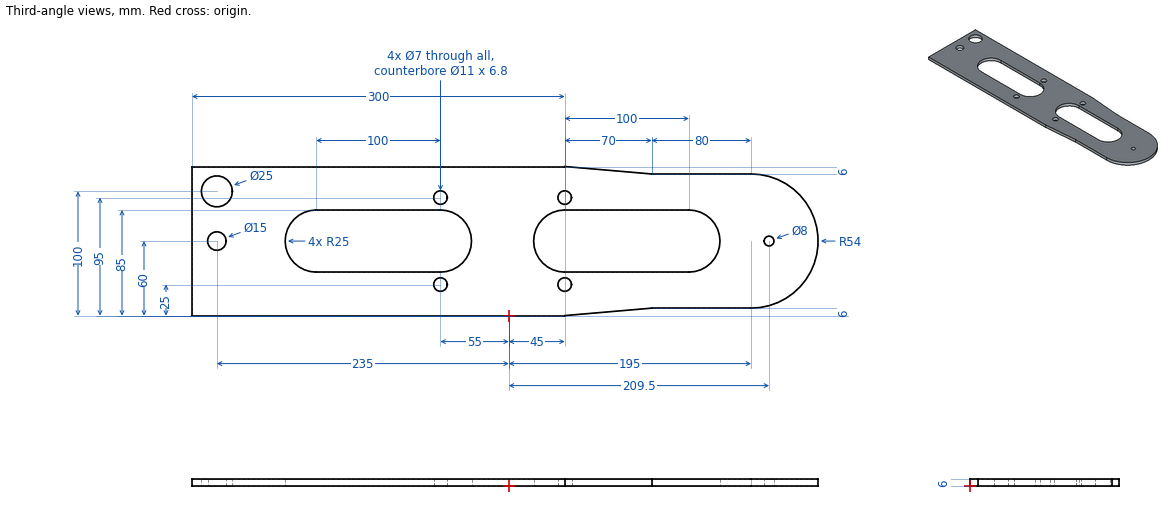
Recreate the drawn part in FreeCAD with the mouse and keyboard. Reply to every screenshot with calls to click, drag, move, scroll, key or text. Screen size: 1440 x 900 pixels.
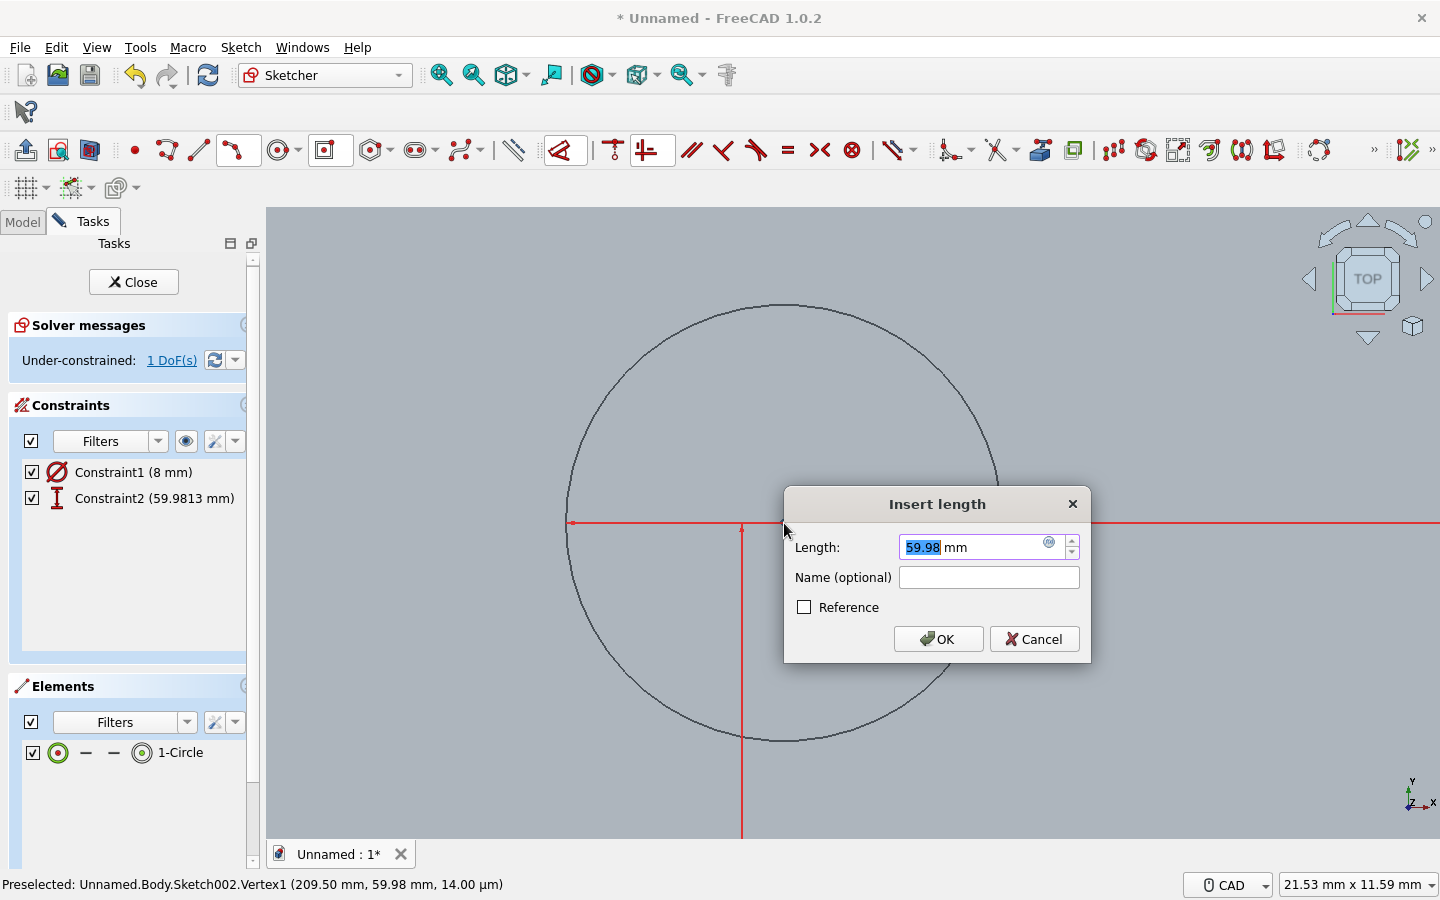
text(60)
key(Return)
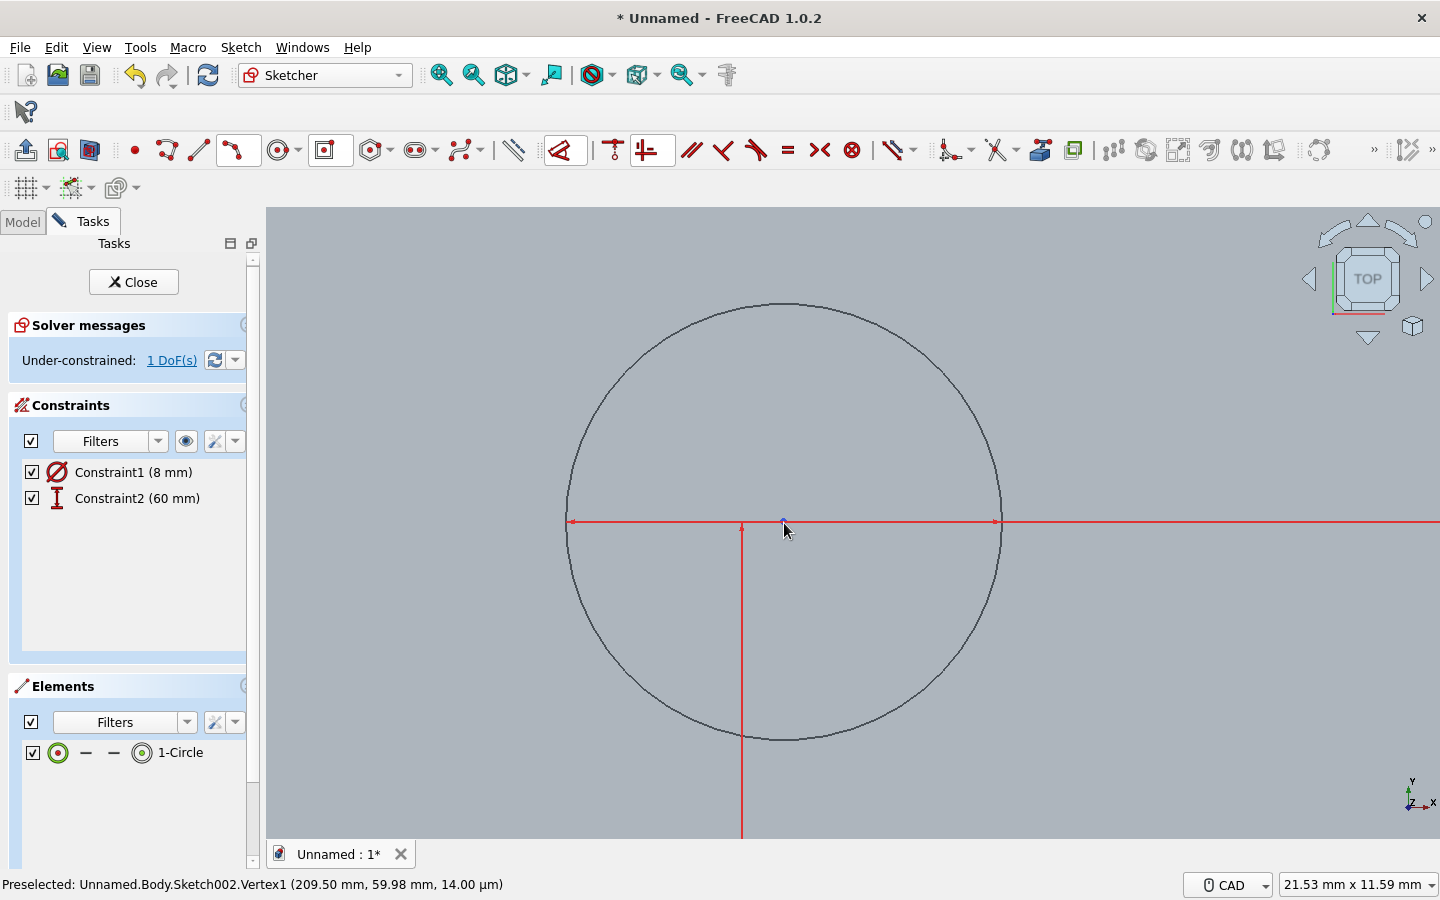
click(784, 522)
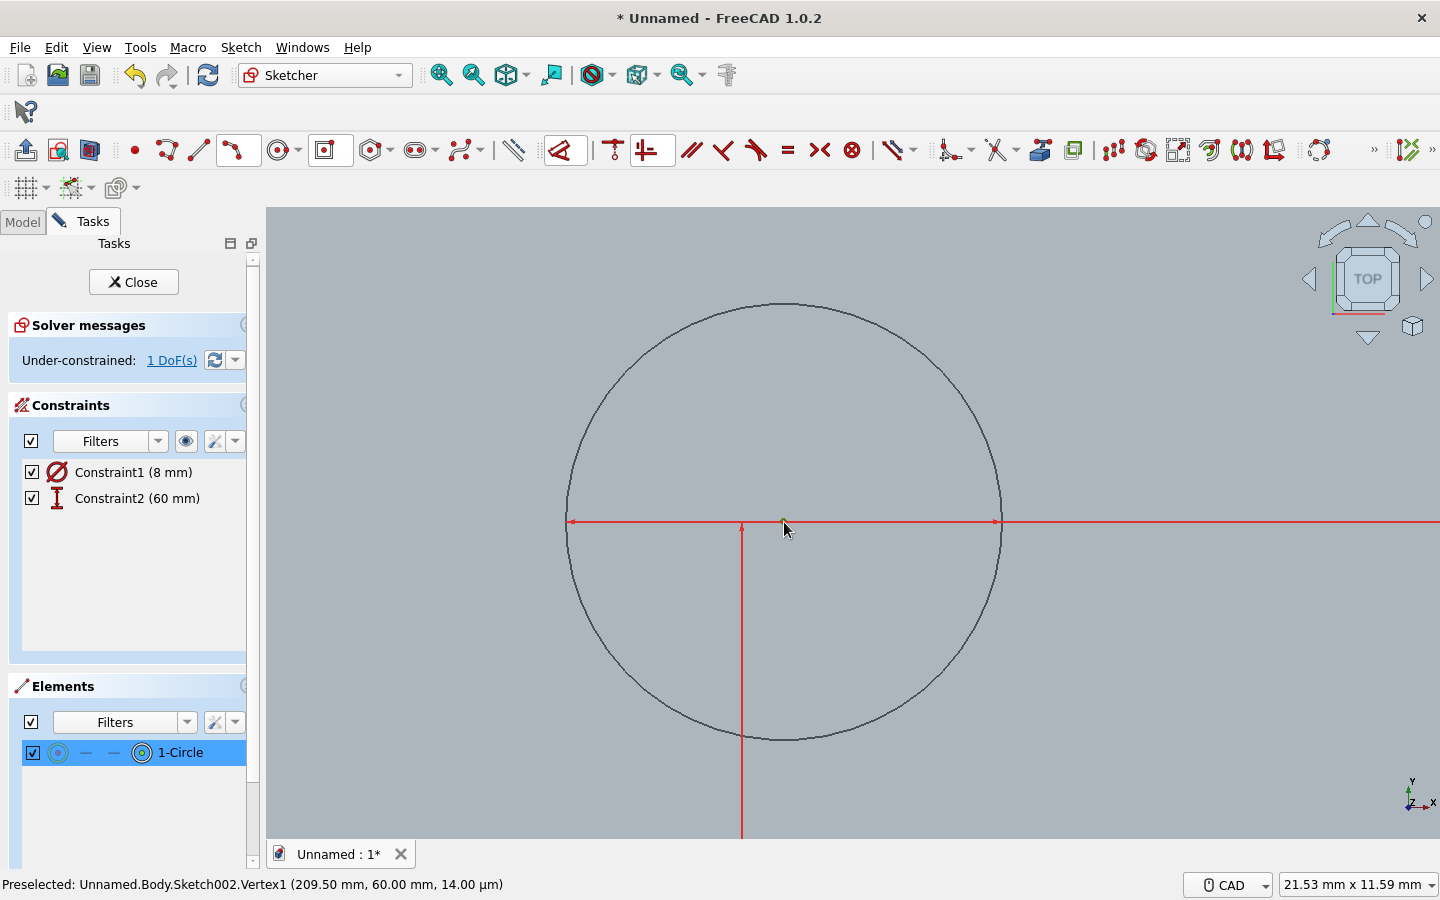
key(l)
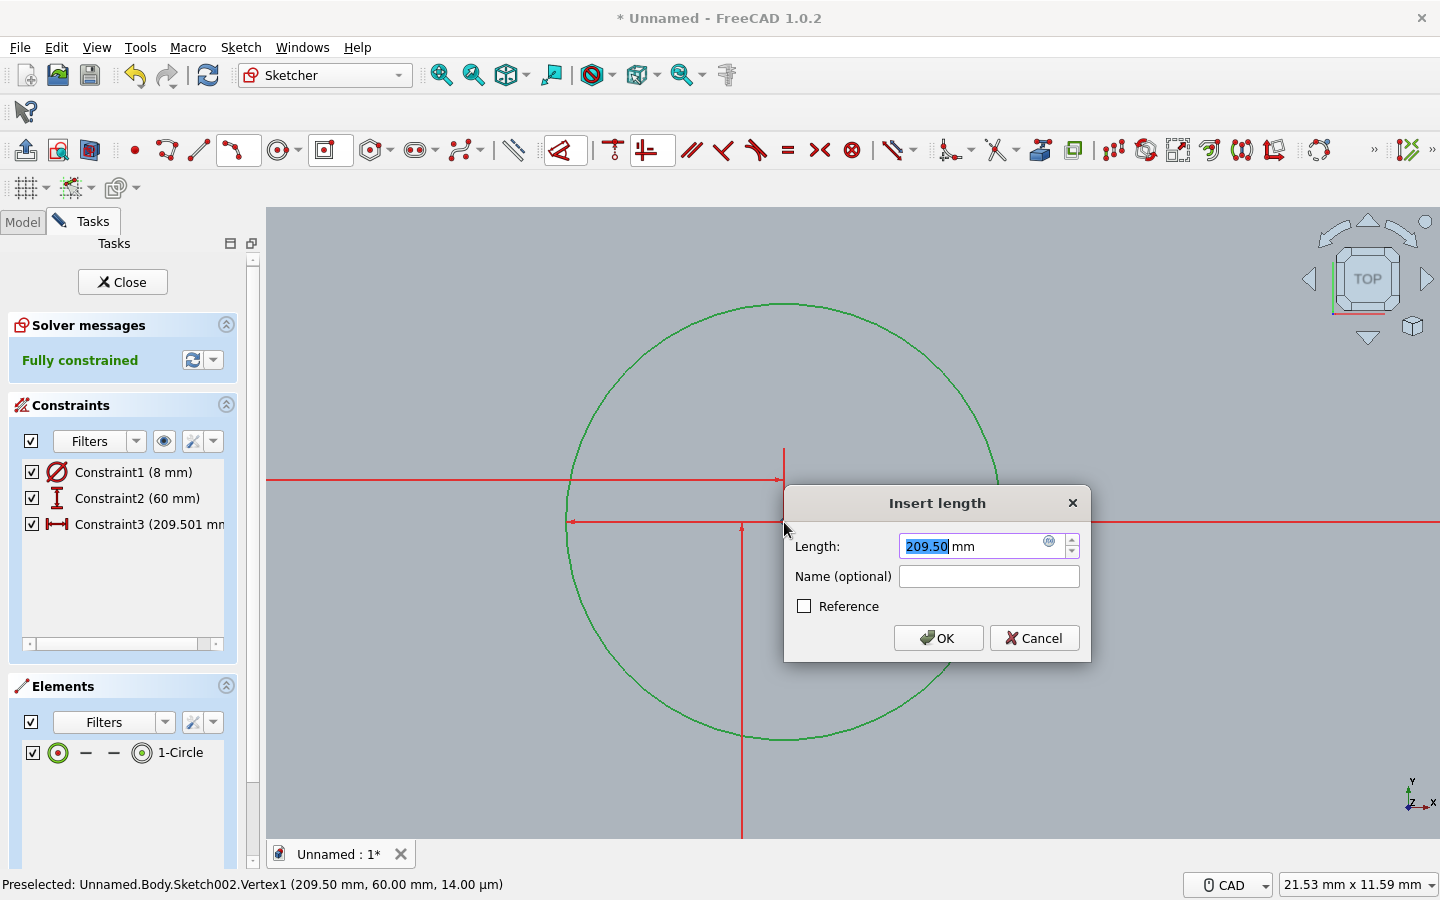
text(209.5)
key(Return)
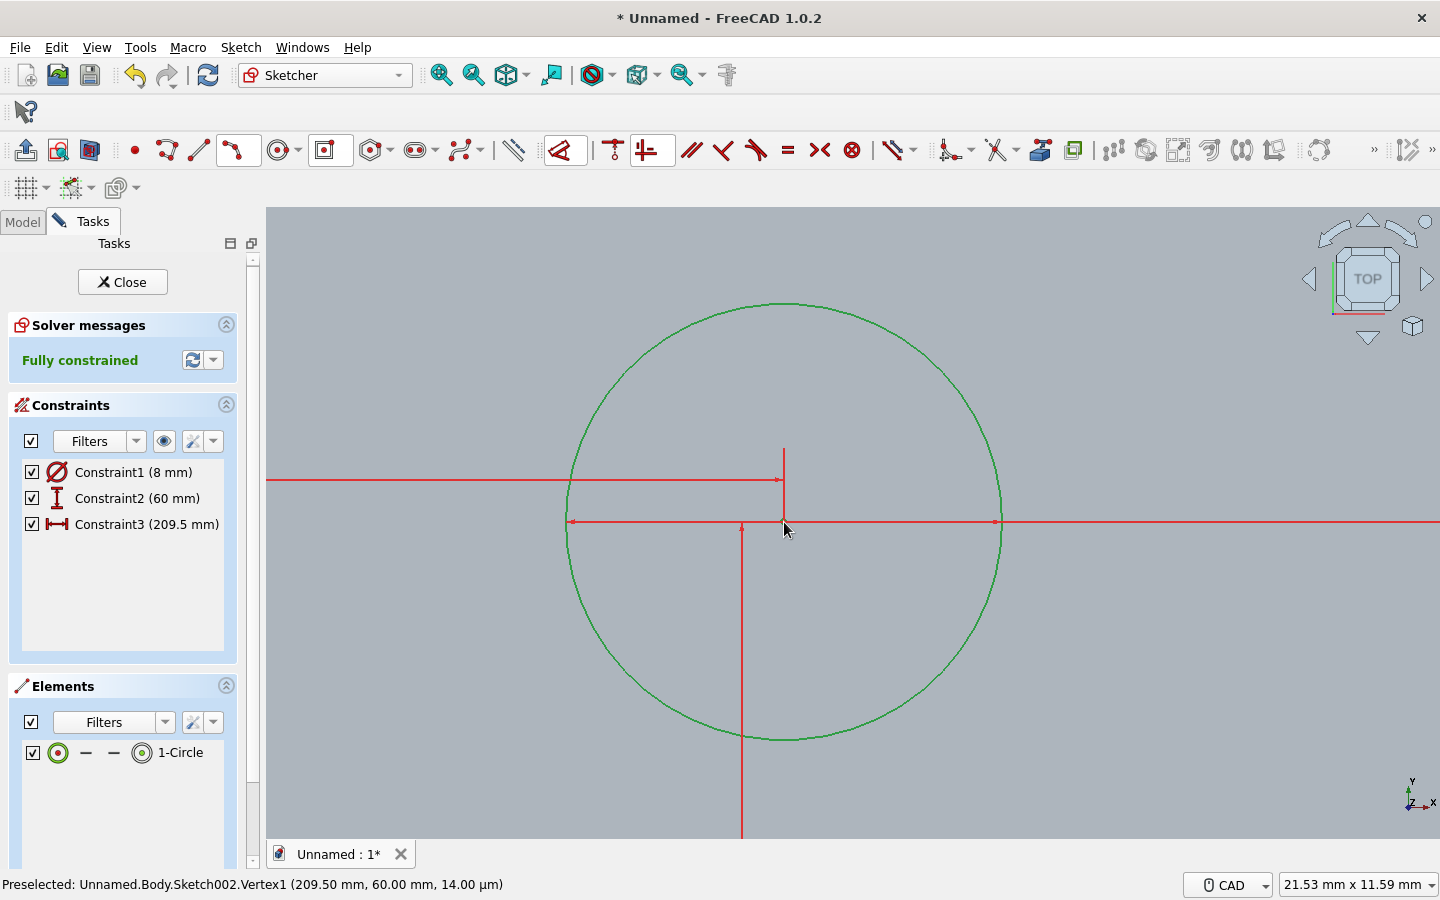
click(123, 282)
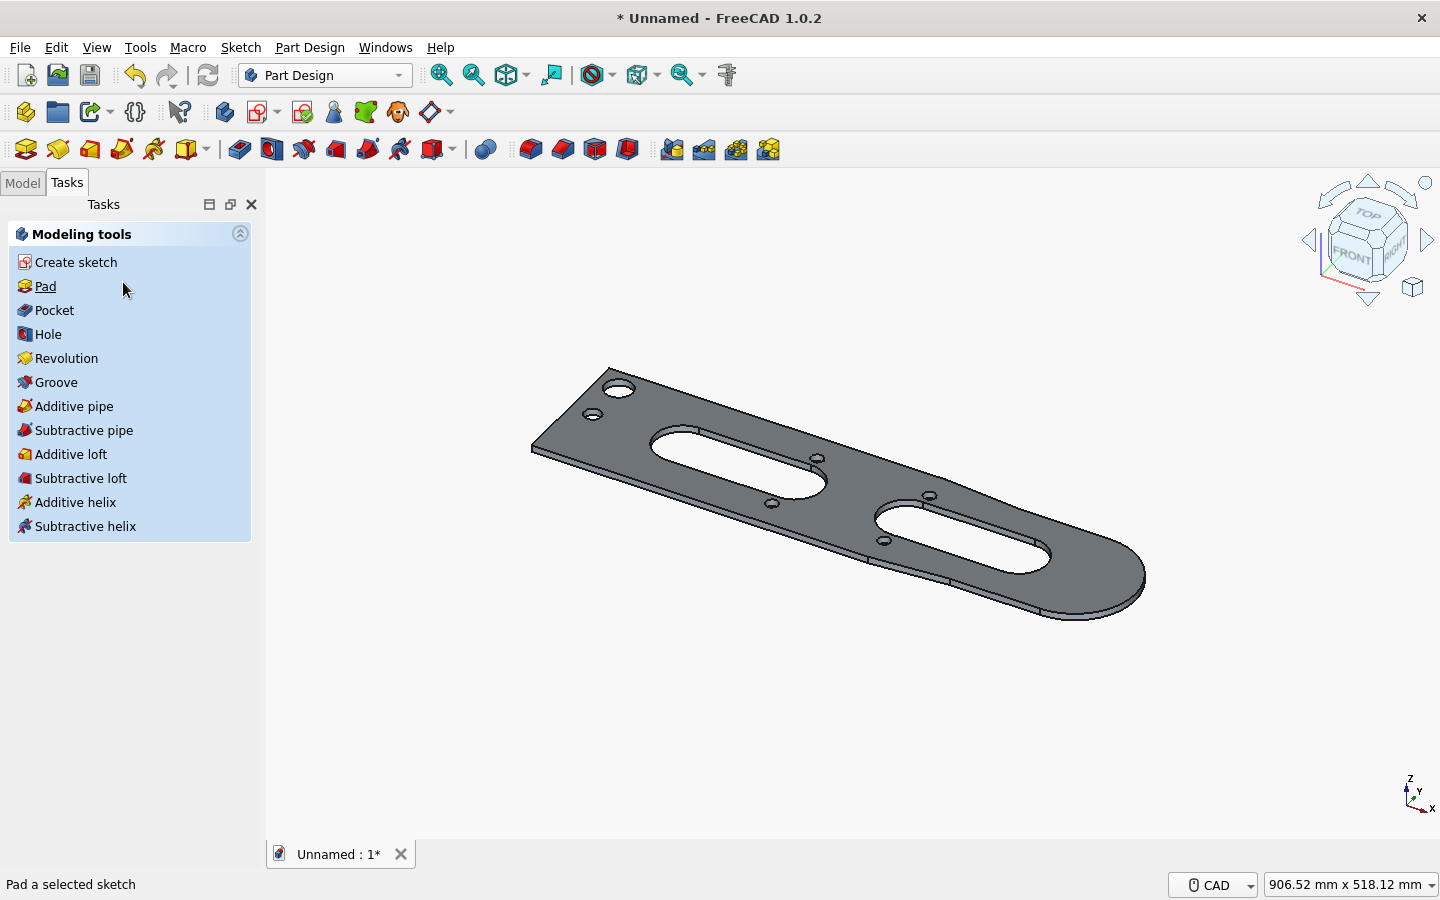
click(240, 150)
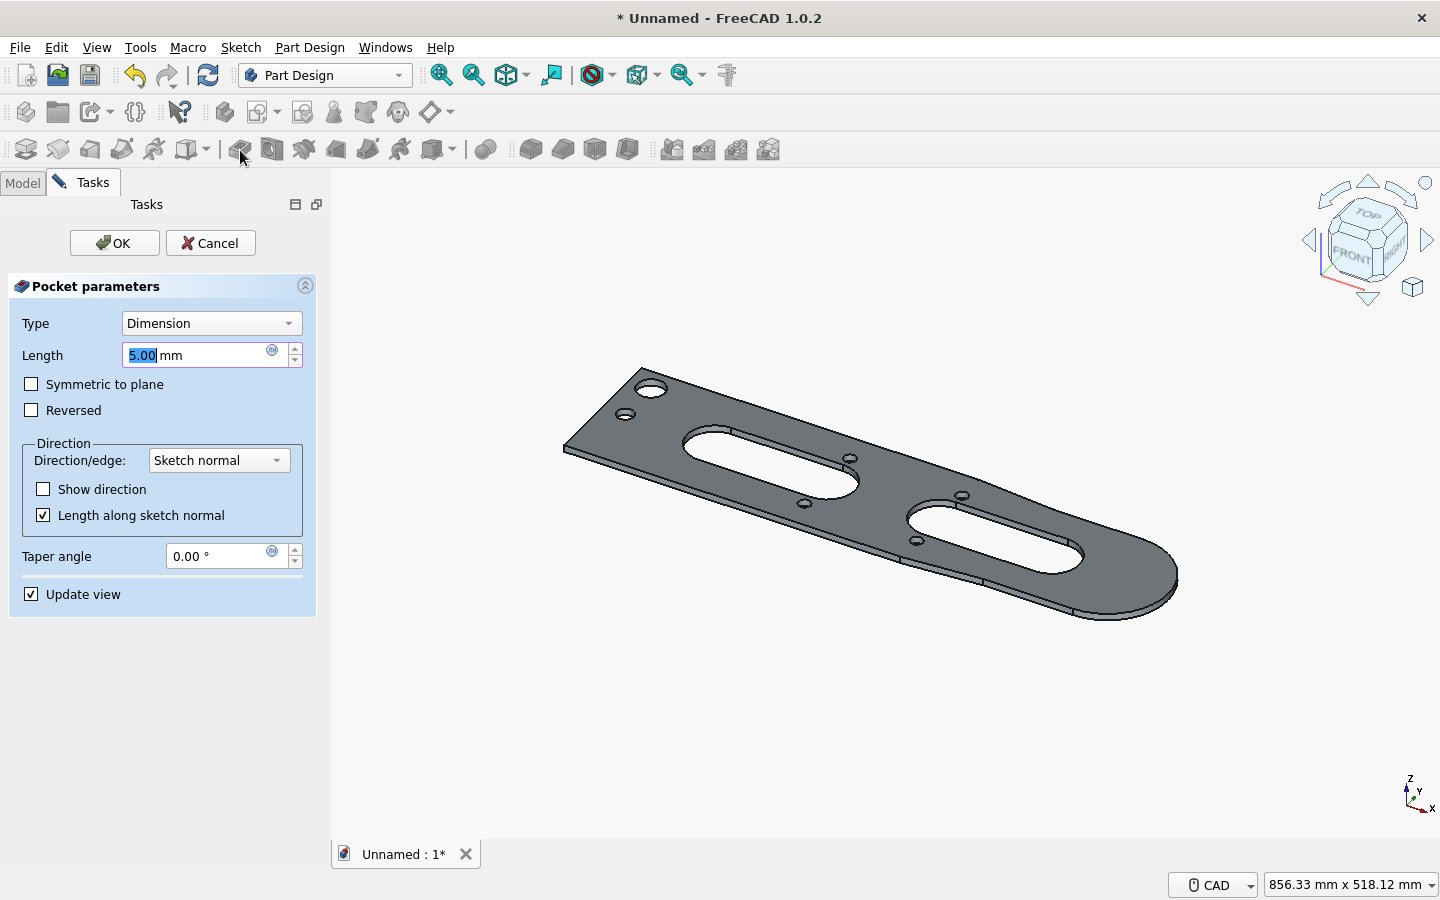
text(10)
key(Tab)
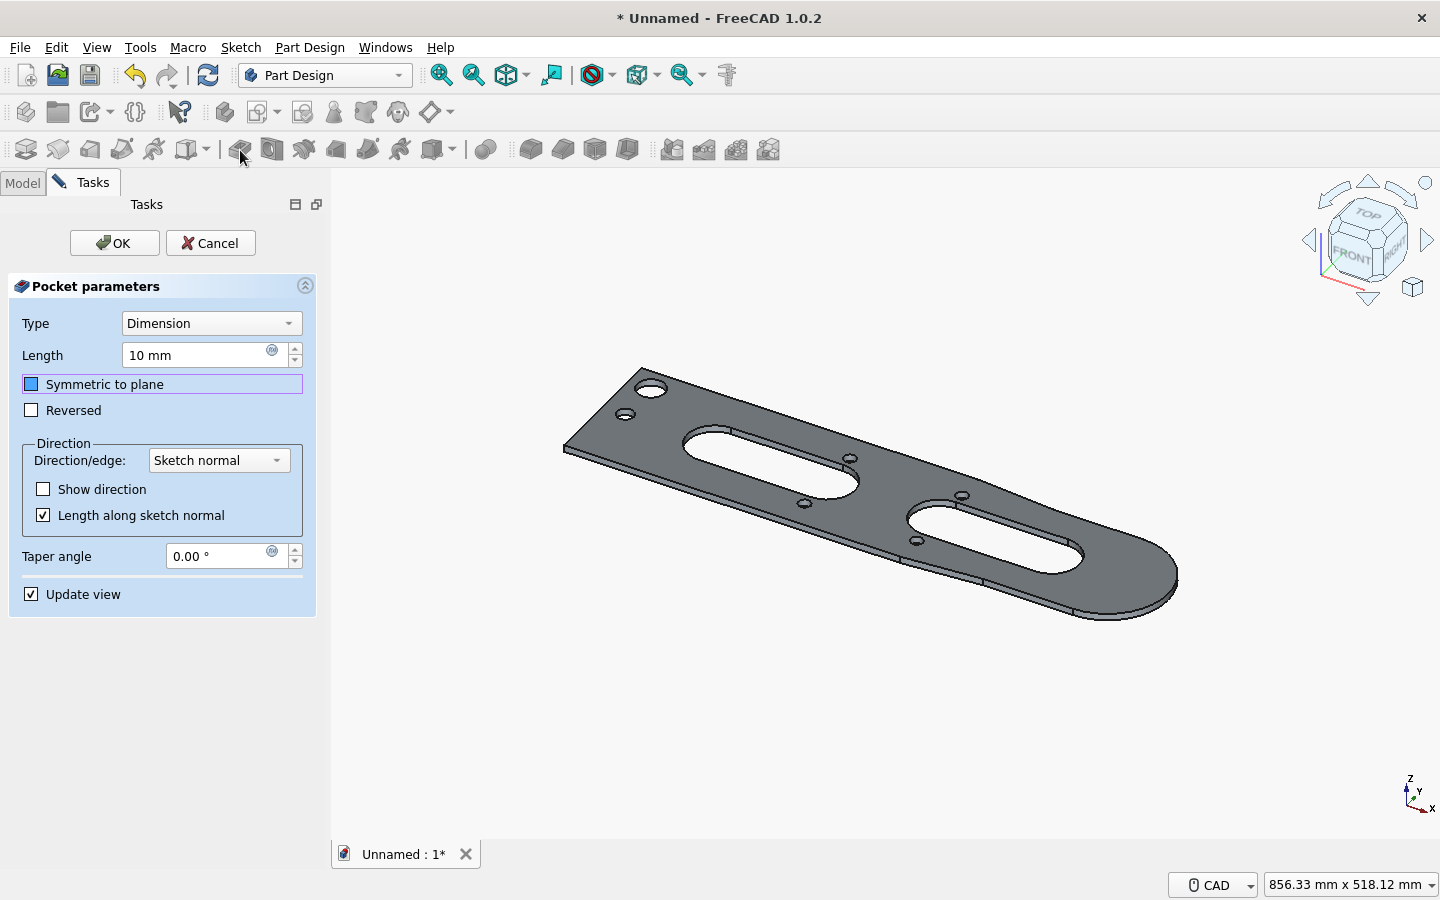
click(30, 410)